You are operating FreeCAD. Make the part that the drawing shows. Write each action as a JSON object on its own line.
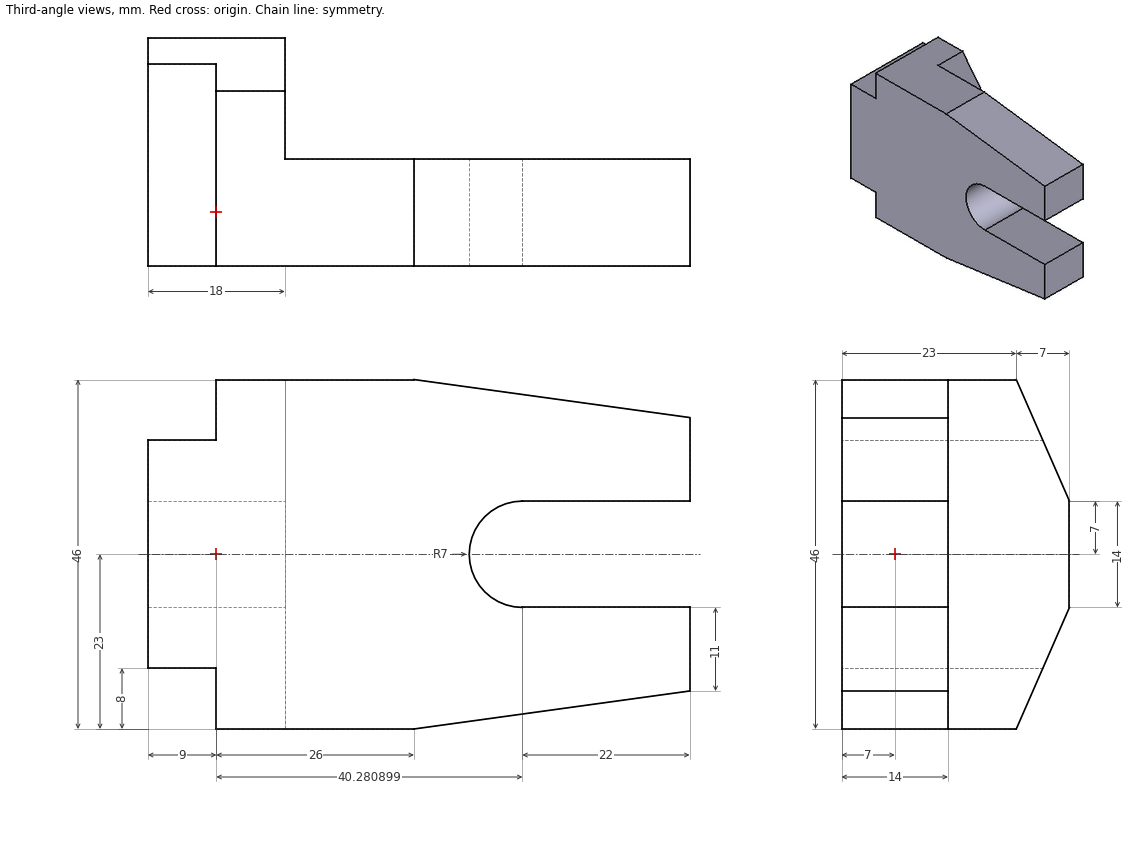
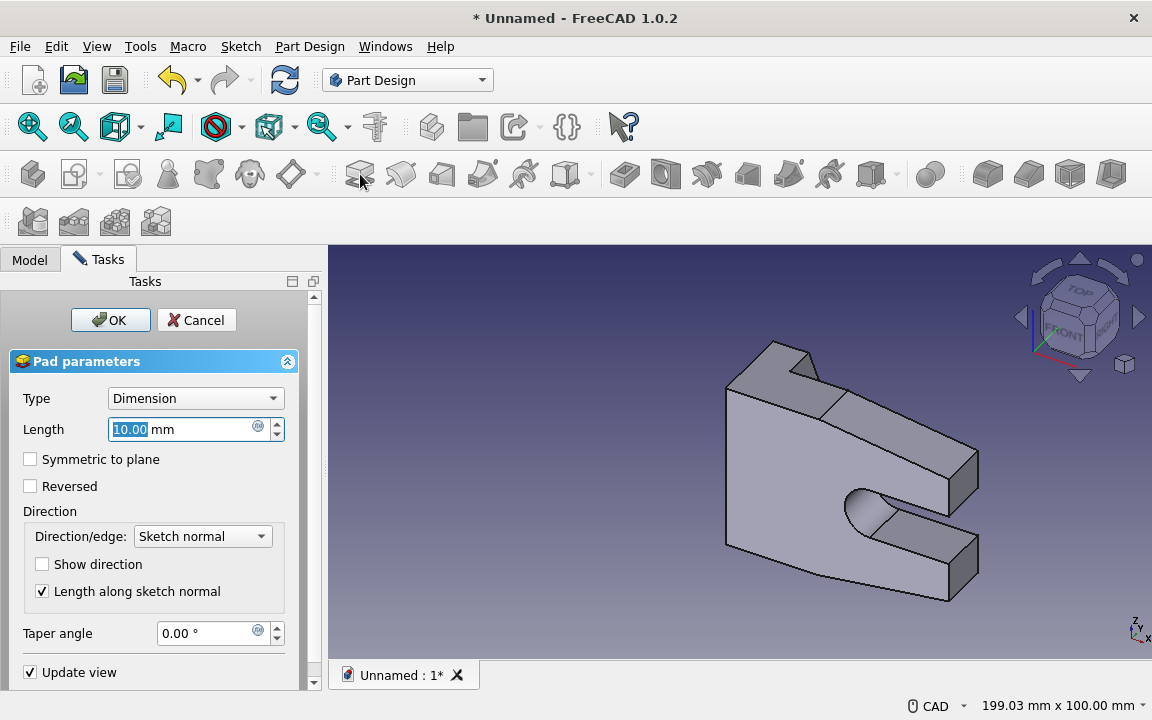
{"action": "type", "text": "18"}
{"action": "key", "text": "Tab"}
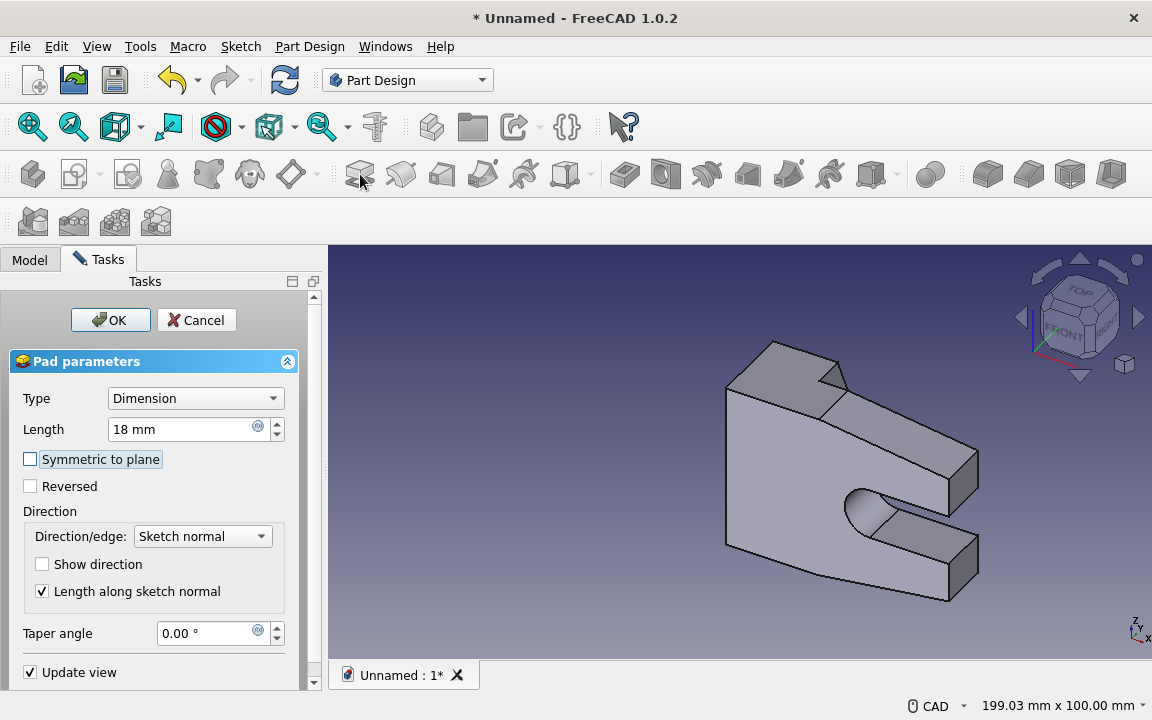
{"action": "left_click", "coordinate": [31, 459]}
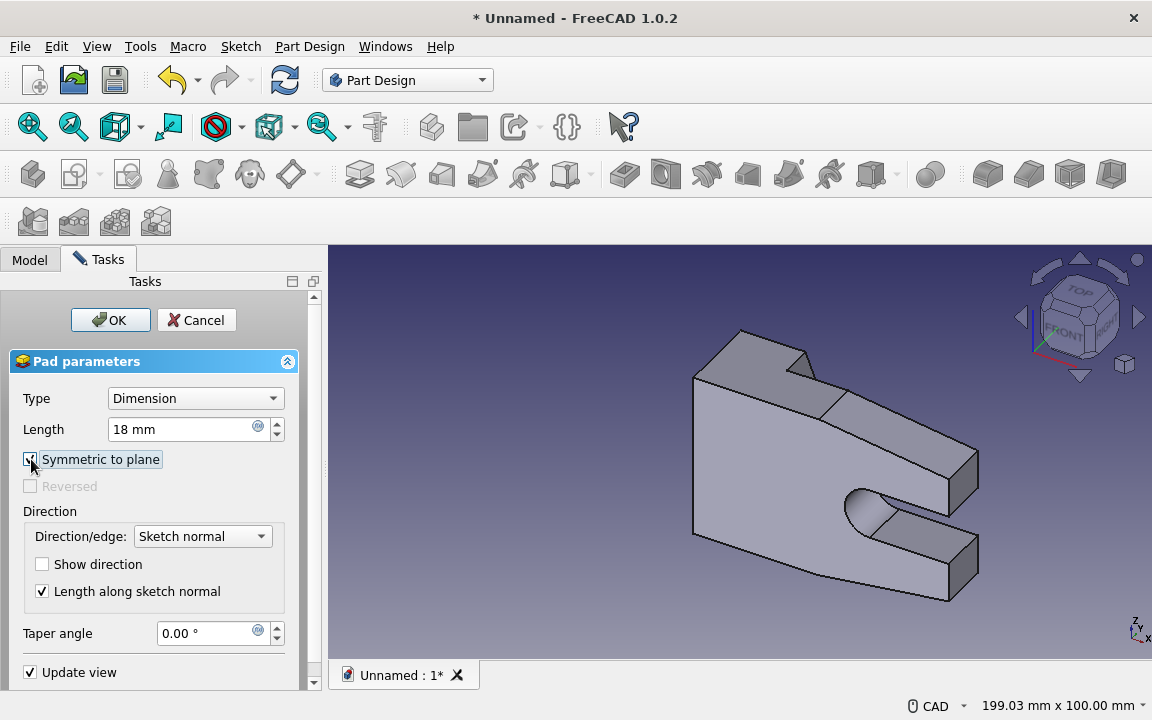
{"action": "left_click", "coordinate": [111, 320]}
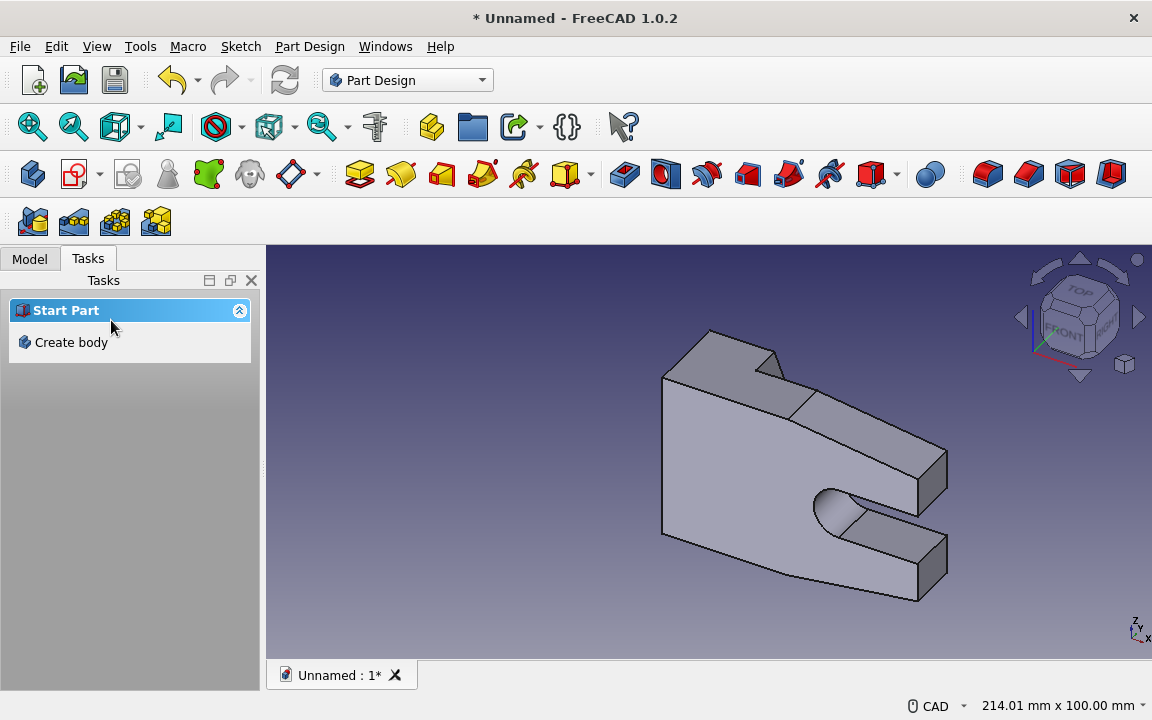
{"action": "key", "text": "4"}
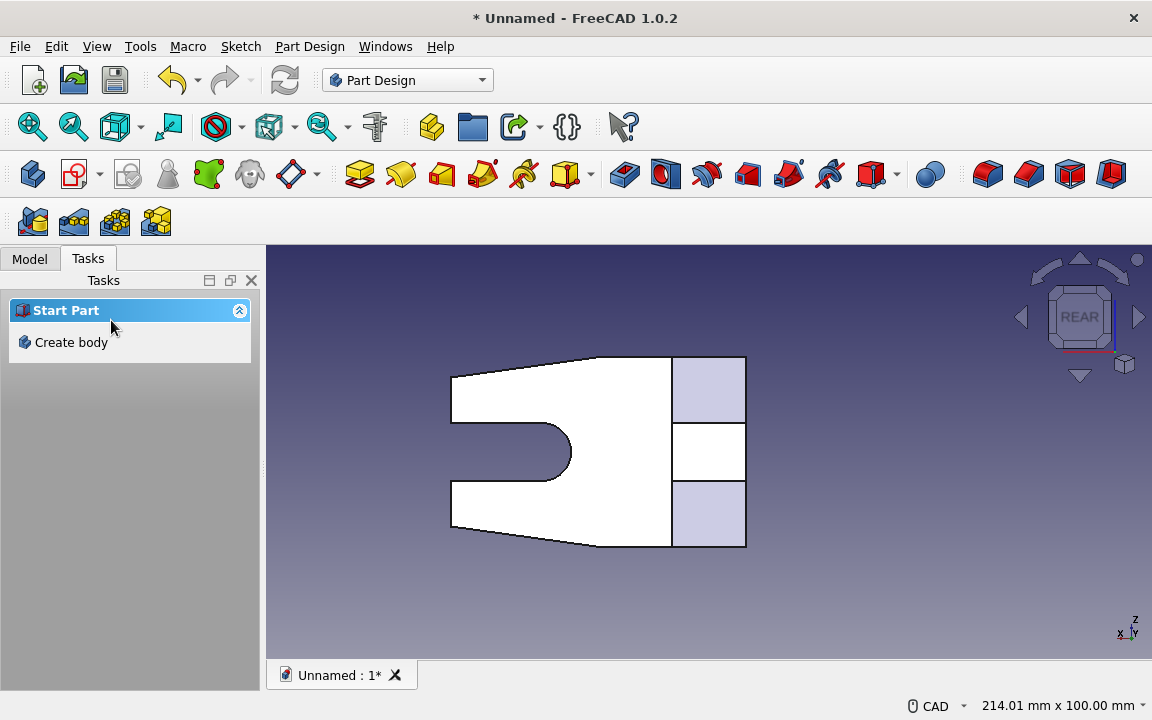
{"action": "left_click", "coordinate": [709, 451]}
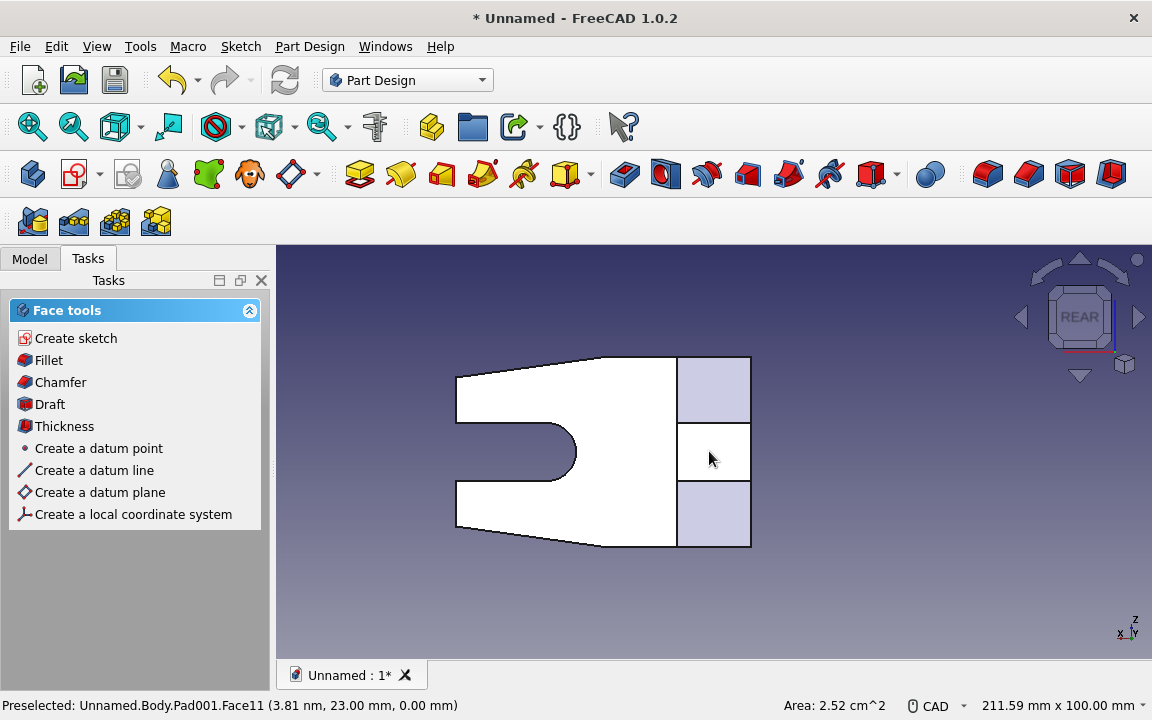
{"action": "left_click", "coordinate": [74, 174]}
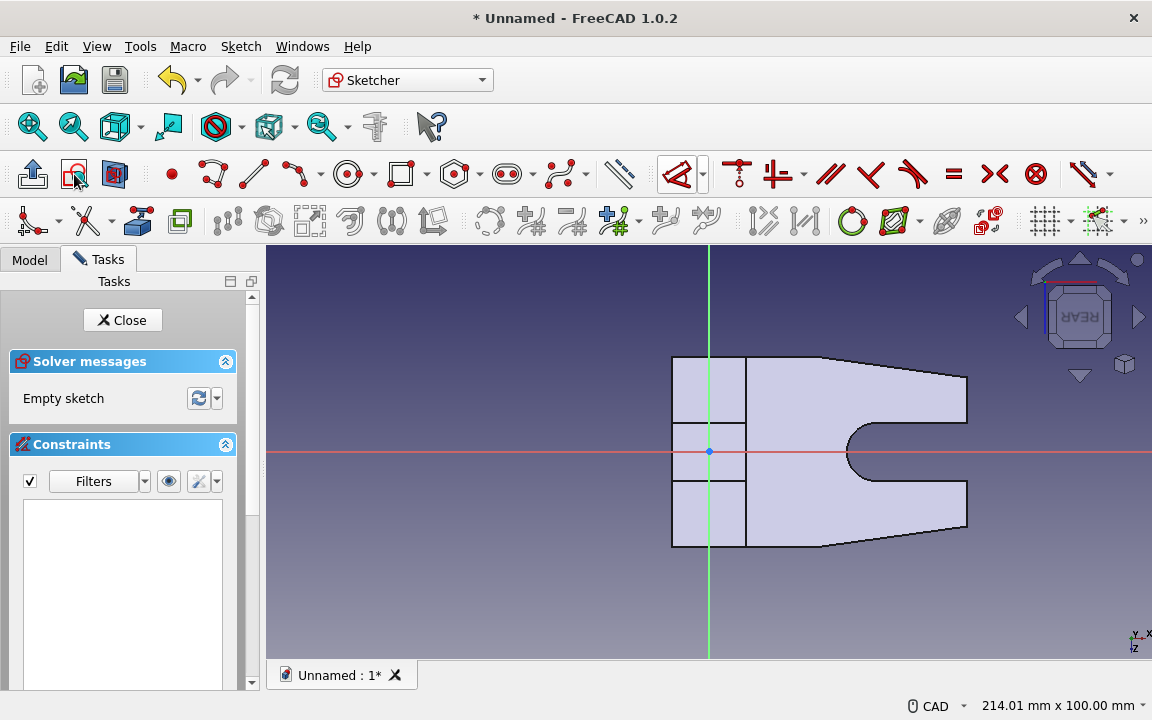
{"action": "key", "text": "g r"}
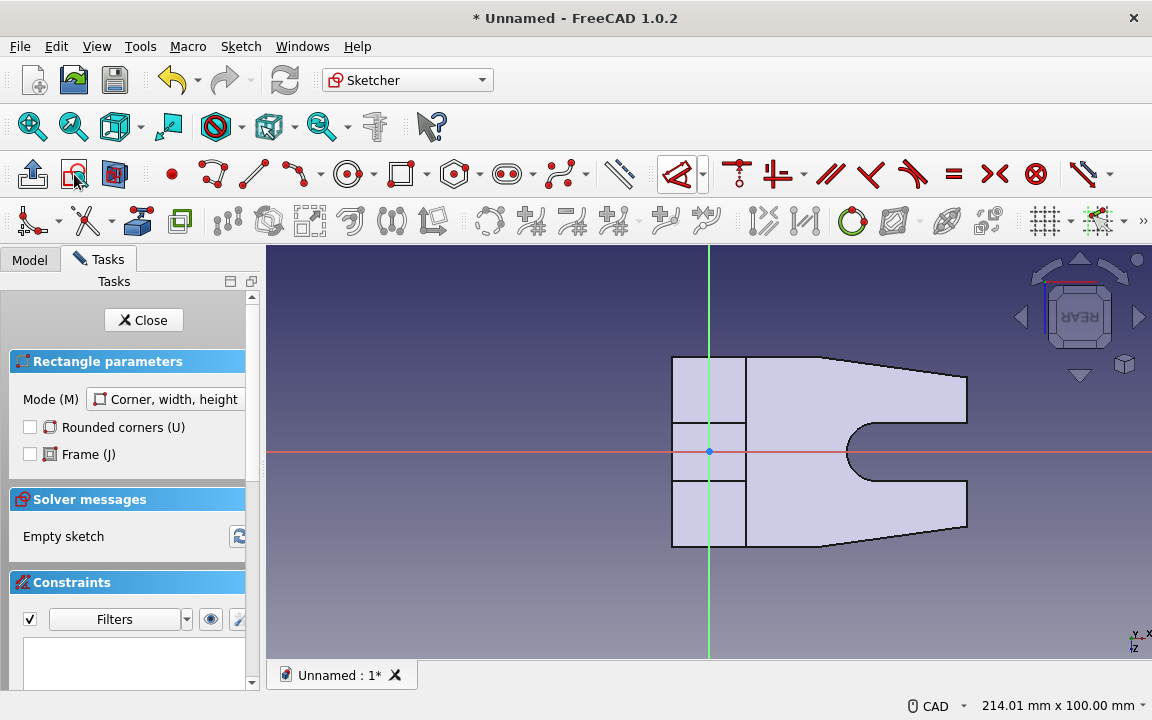
{"action": "left_click", "coordinate": [672, 357]}
{"action": "left_click", "coordinate": [709, 390]}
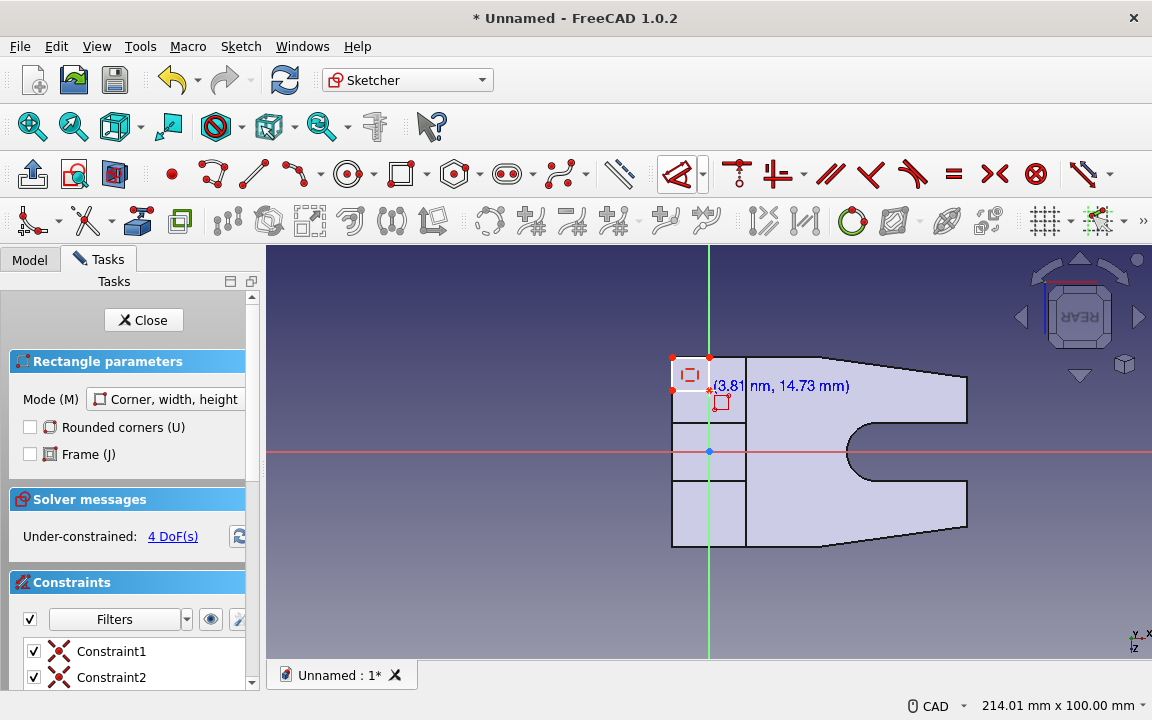
{"action": "left_click", "coordinate": [672, 514]}
{"action": "left_click", "coordinate": [709, 547]}
{"action": "key", "text": "Escape"}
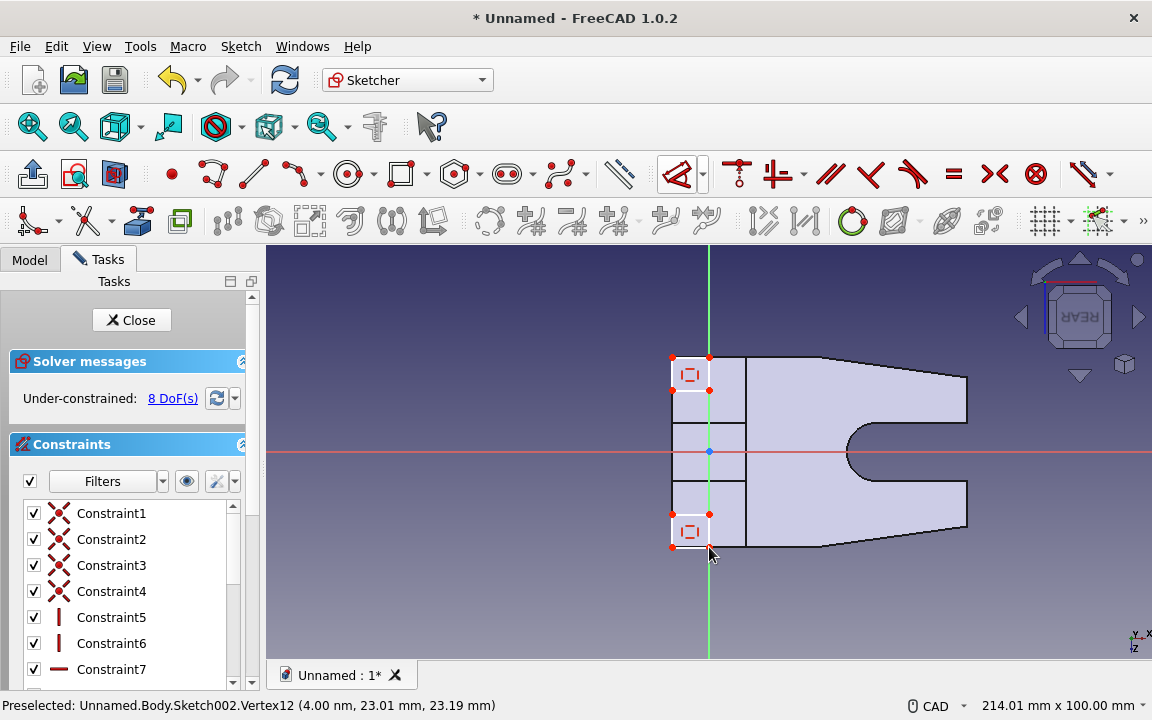
{"action": "left_click", "coordinate": [672, 391]}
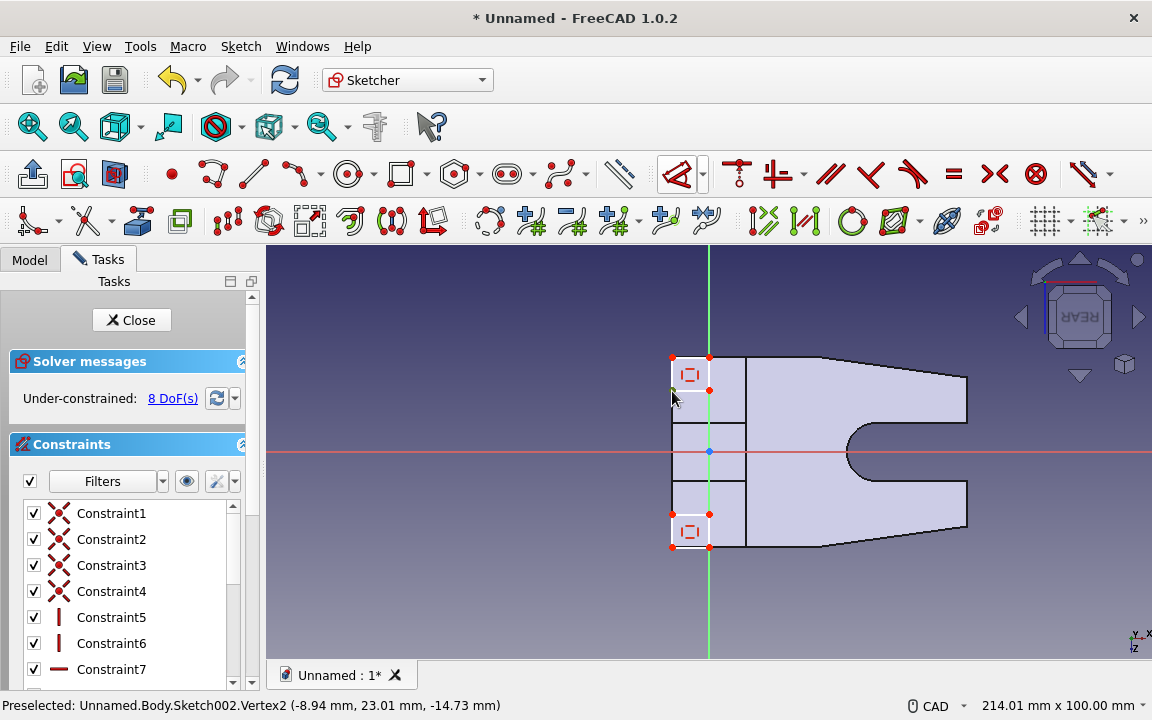
{"action": "left_click", "coordinate": [672, 515]}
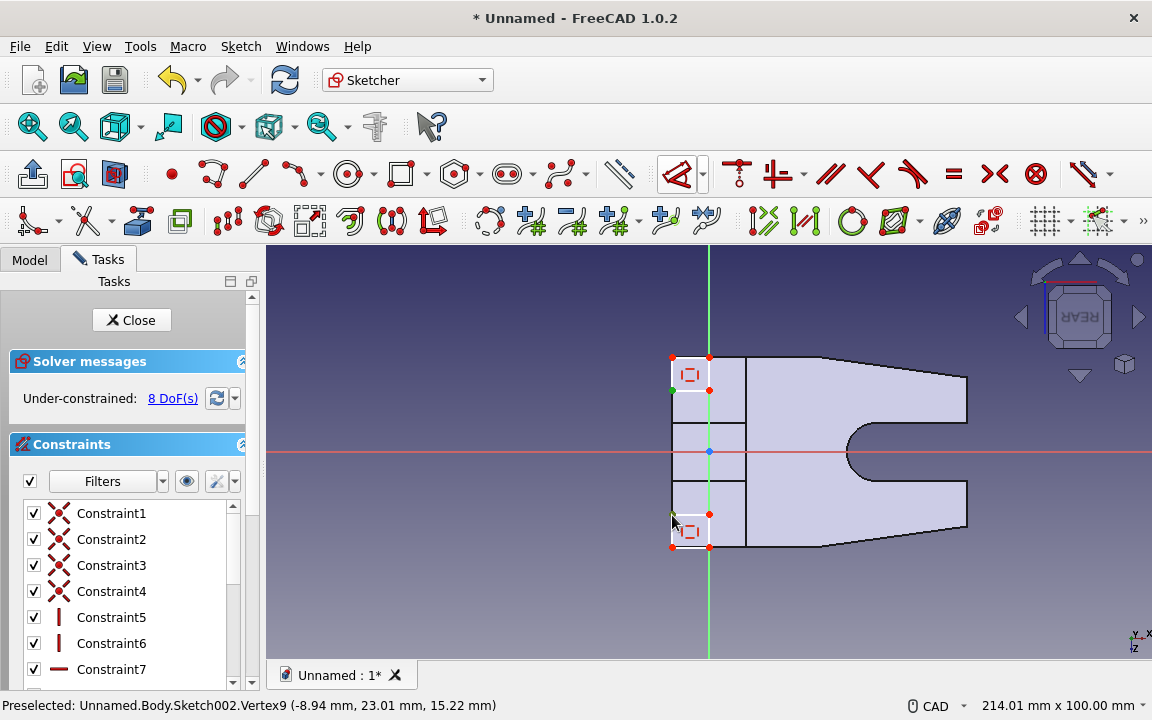
{"action": "left_click", "coordinate": [344, 452]}